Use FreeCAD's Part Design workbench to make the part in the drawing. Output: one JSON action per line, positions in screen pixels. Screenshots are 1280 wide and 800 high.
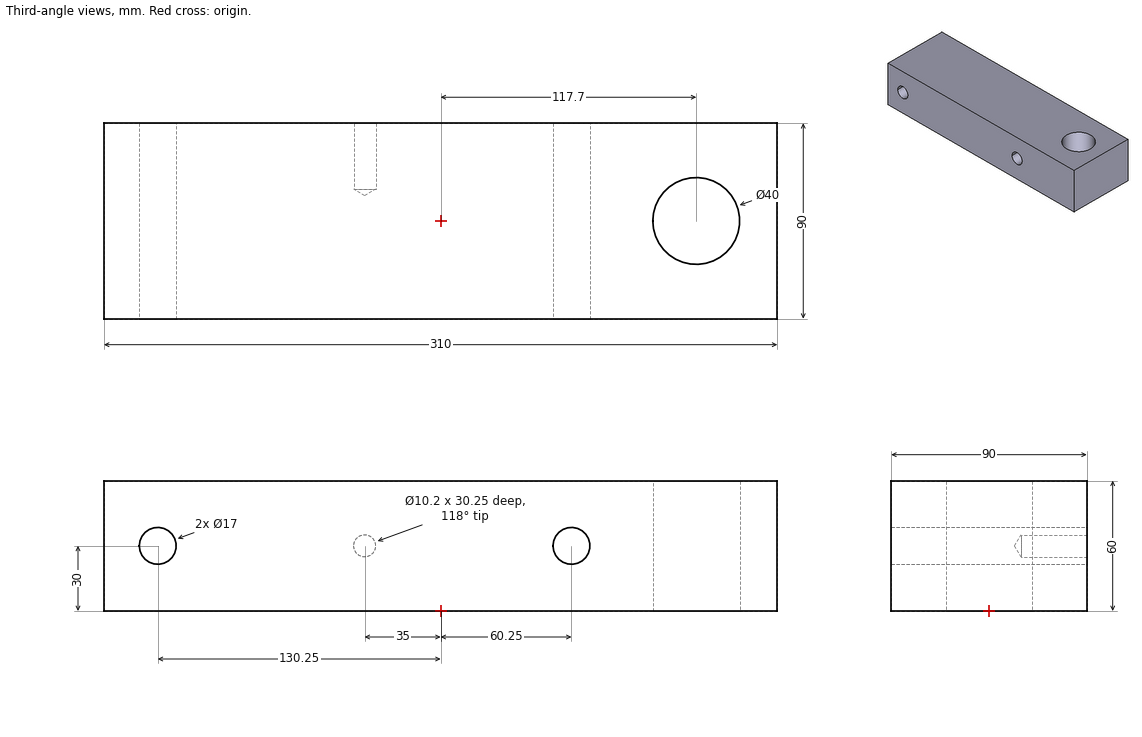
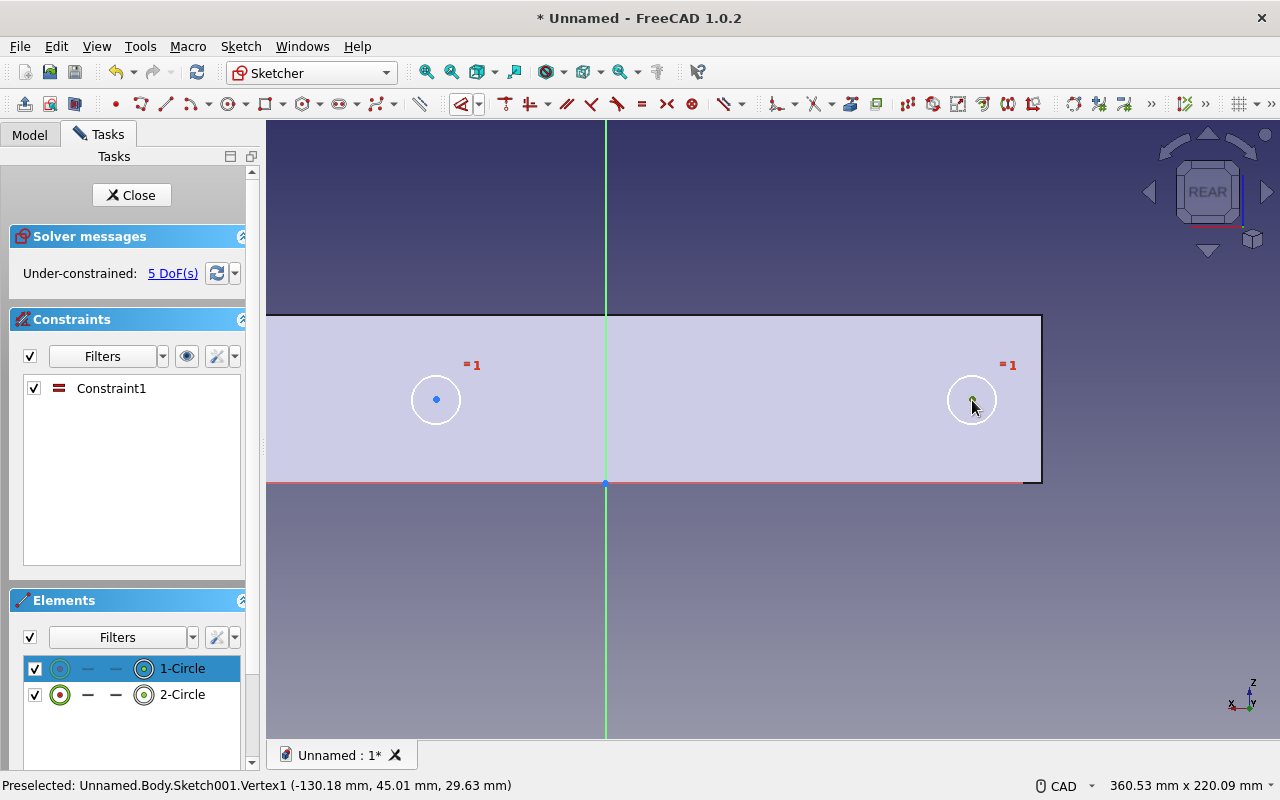
{"action": "left_click", "coordinate": [436, 400]}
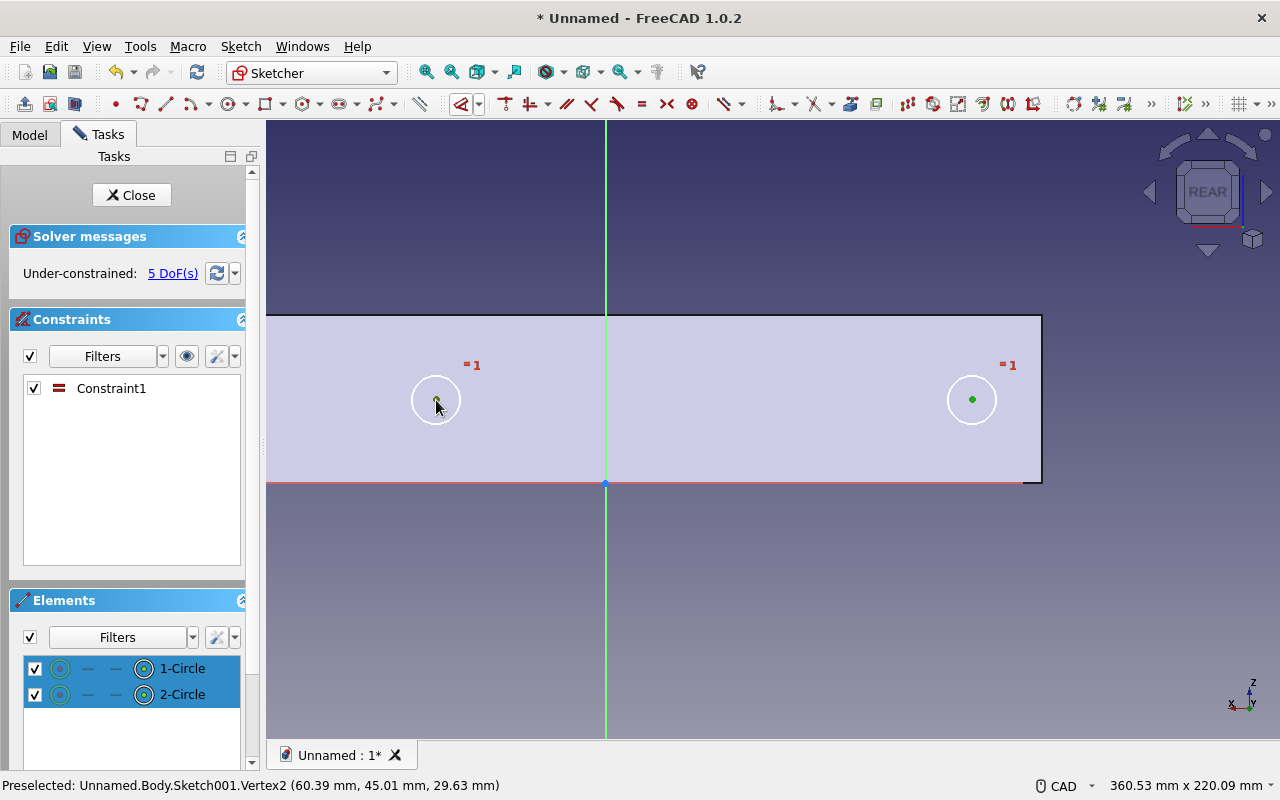
{"action": "key", "text": "h"}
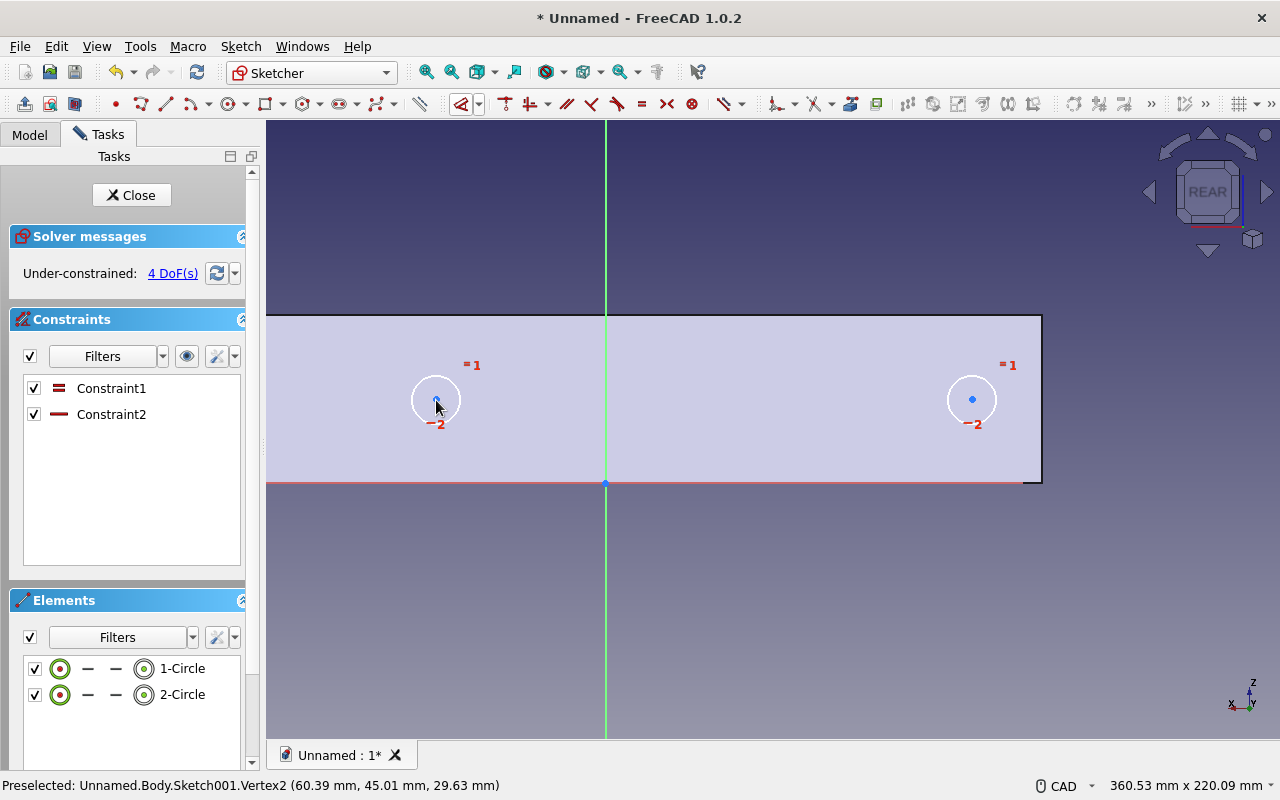
{"action": "left_click", "coordinate": [989, 383]}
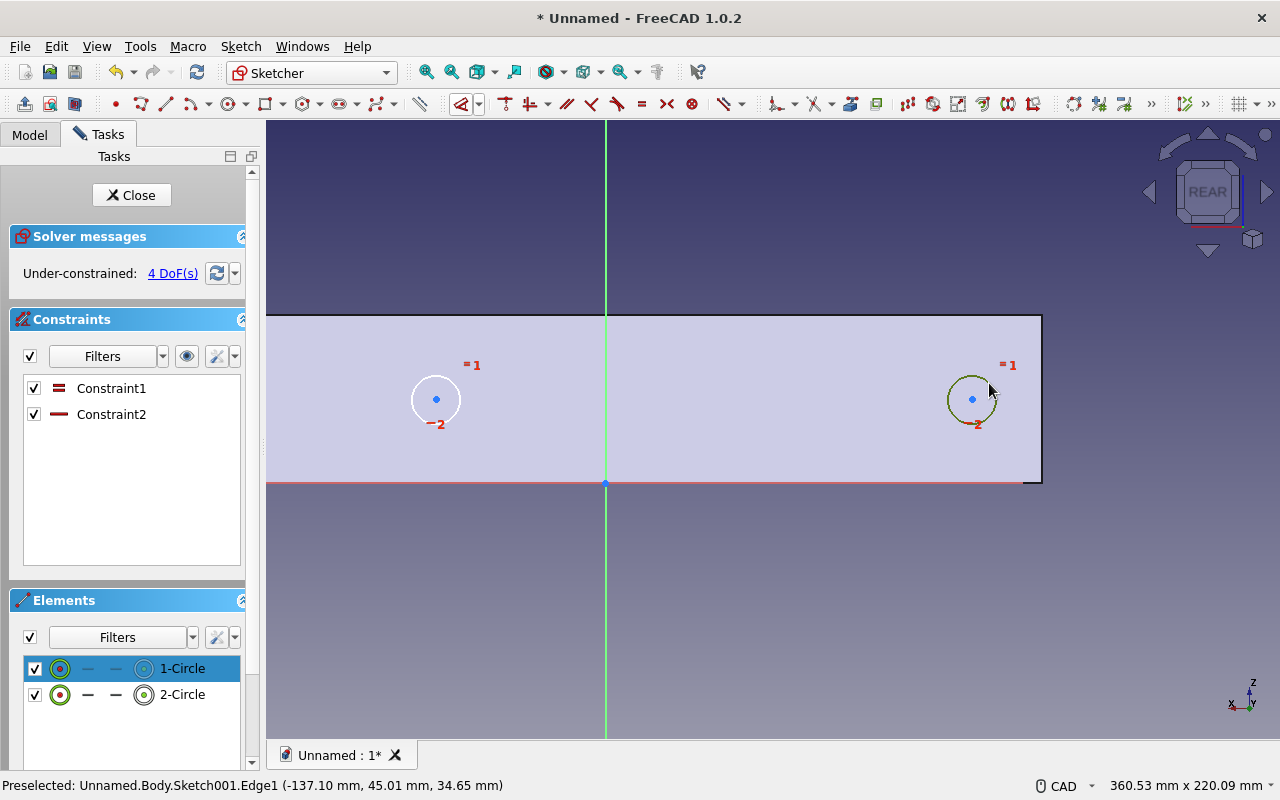
{"action": "left_click", "coordinate": [478, 104]}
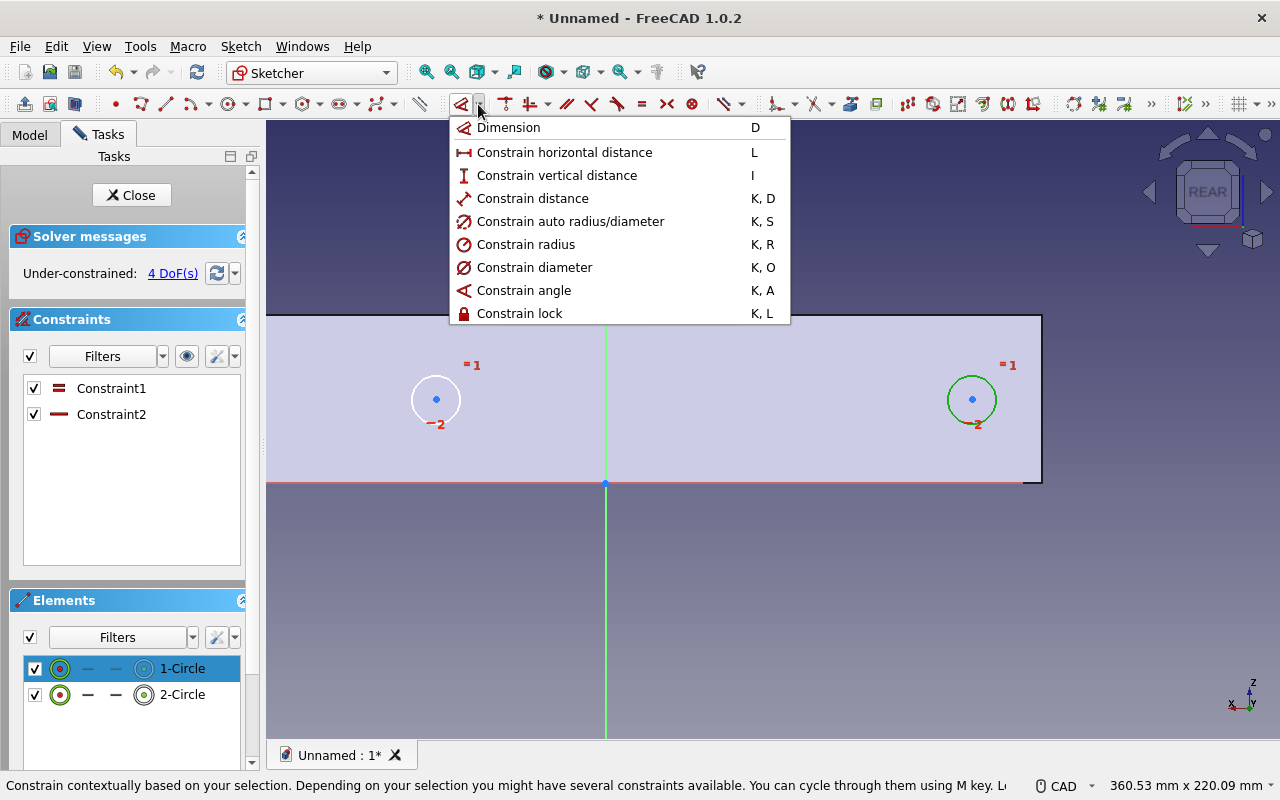
{"action": "left_click", "coordinate": [620, 268]}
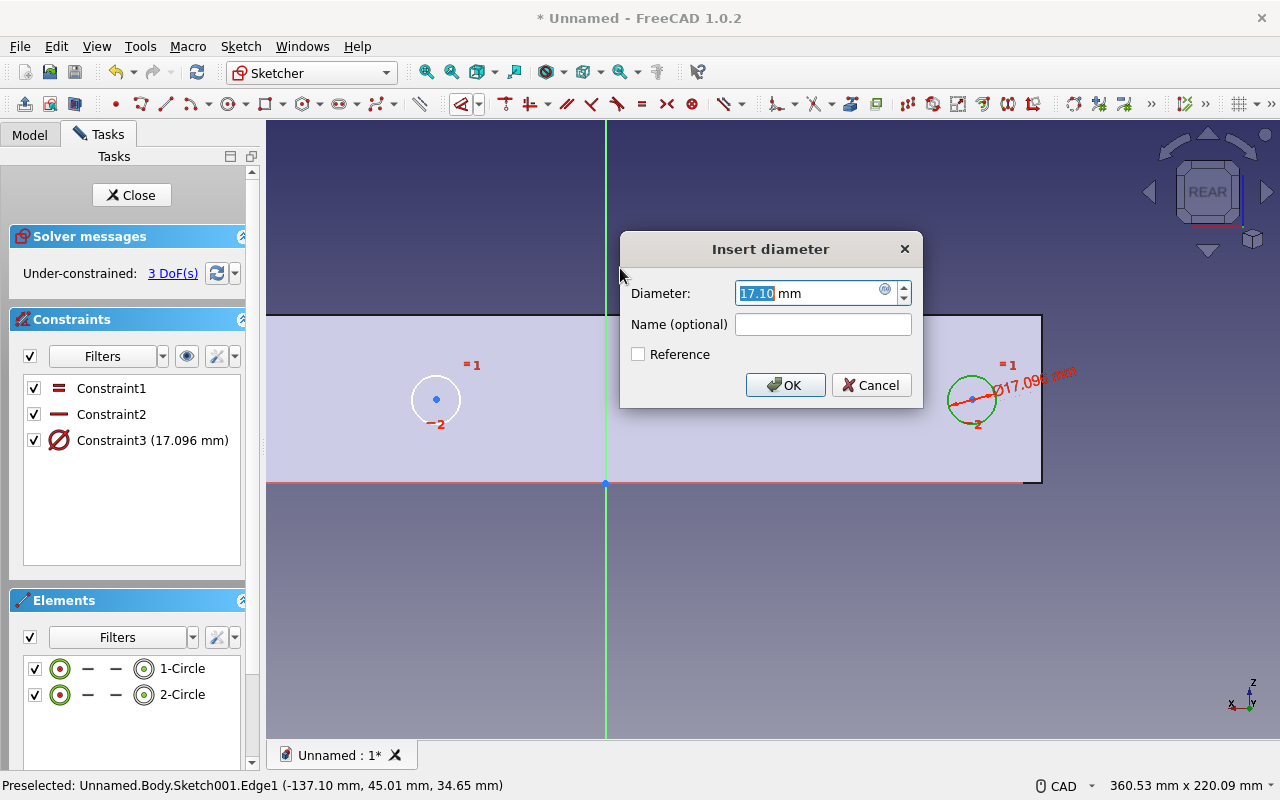
{"action": "type", "text": "17"}
{"action": "key", "text": "Return"}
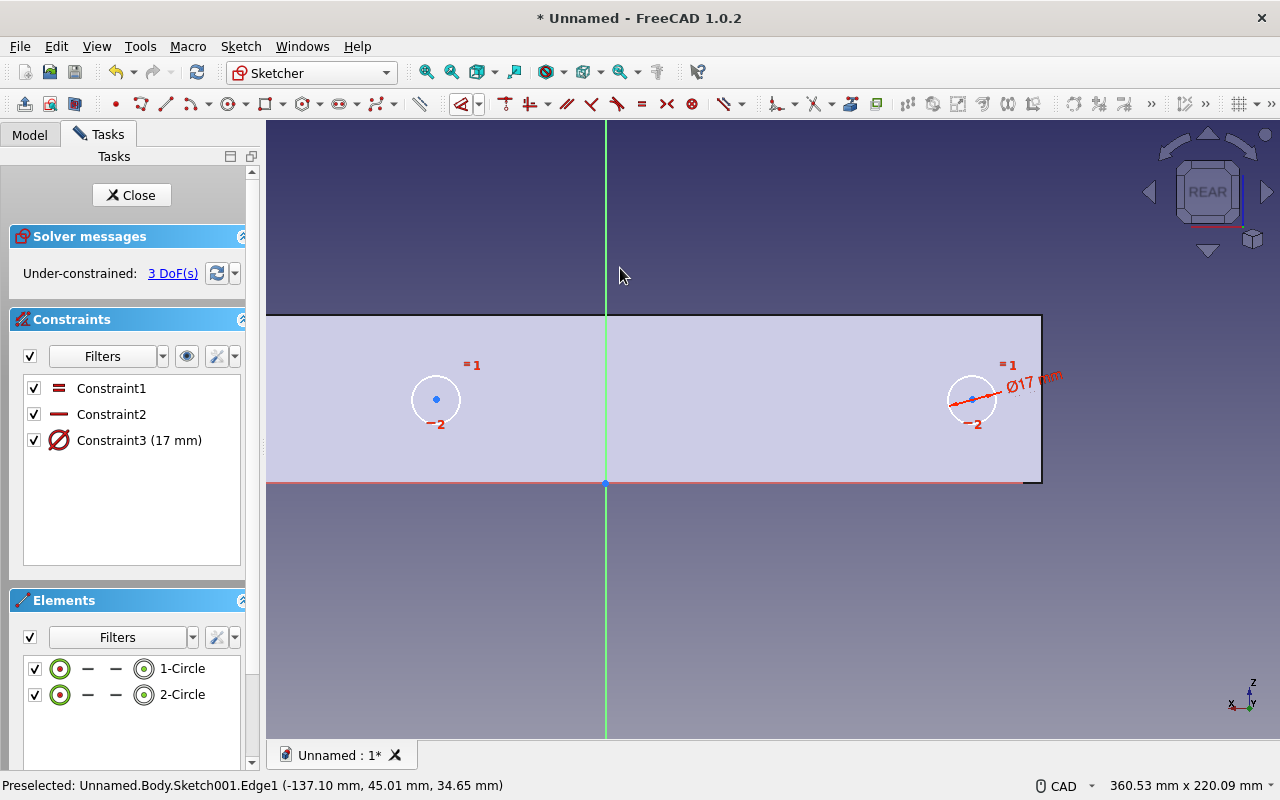
{"action": "left_click", "coordinate": [972, 400]}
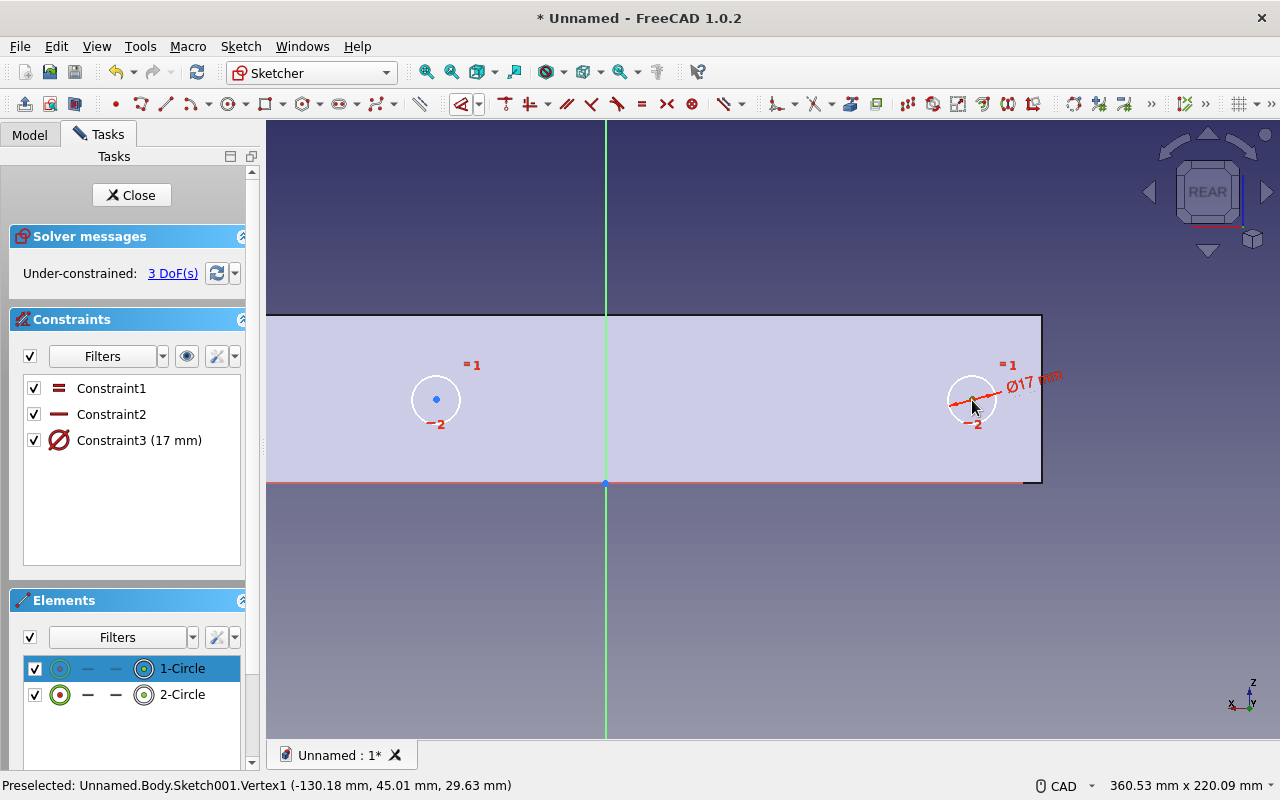
{"action": "key", "text": "i"}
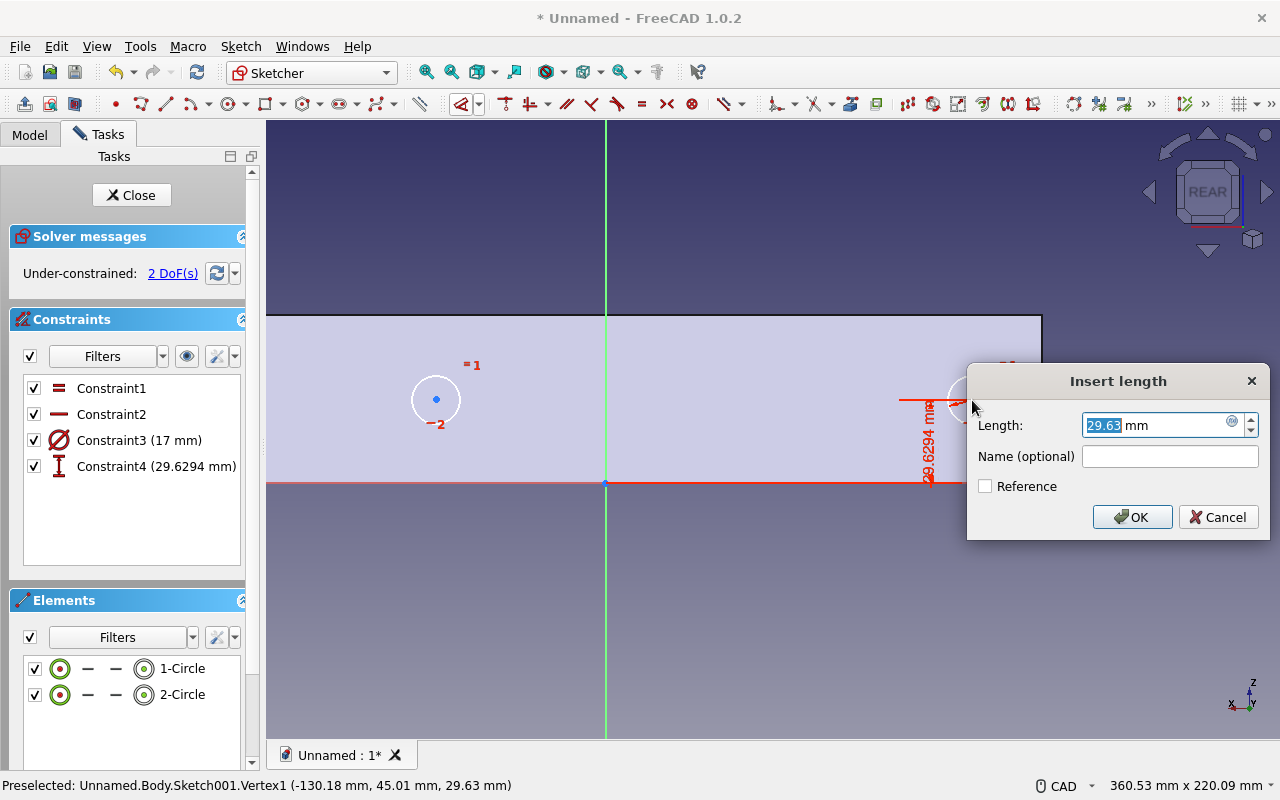
{"action": "type", "text": "30"}
{"action": "key", "text": "Return"}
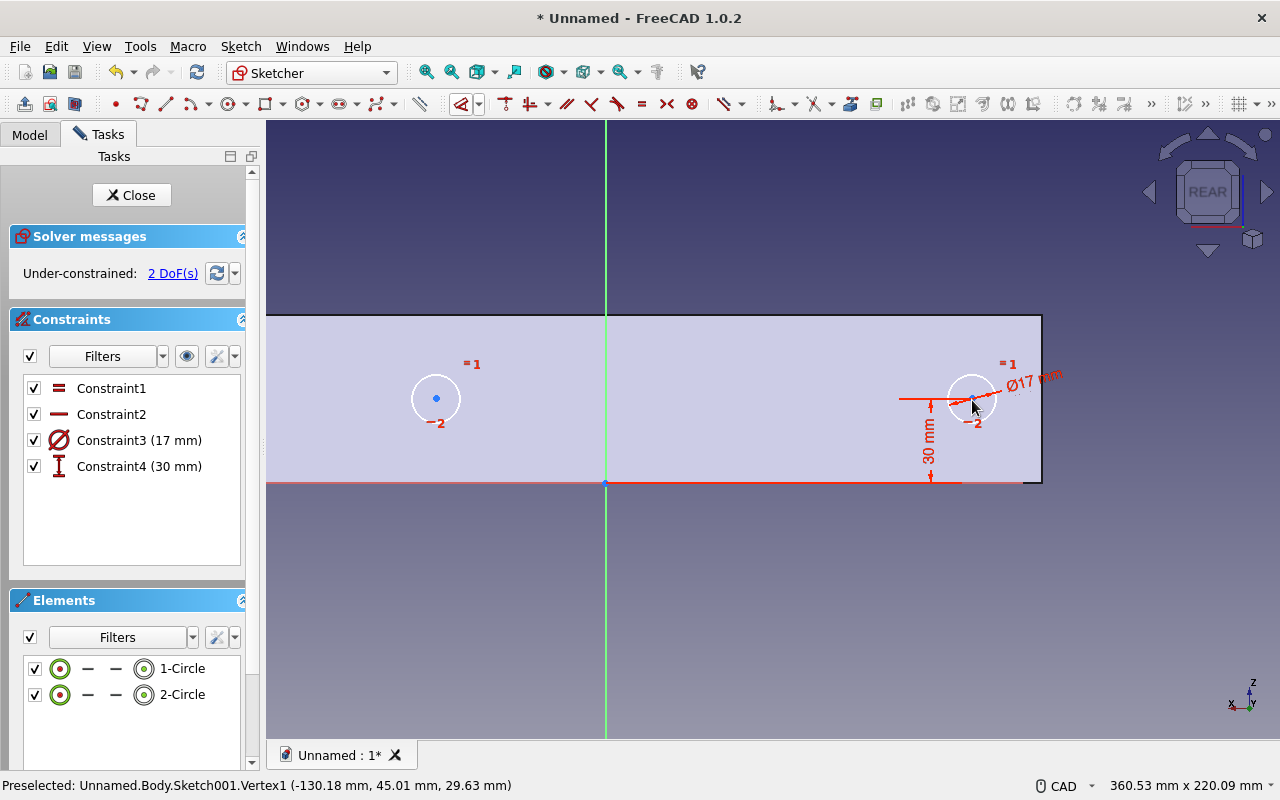
{"action": "left_click", "coordinate": [436, 399]}